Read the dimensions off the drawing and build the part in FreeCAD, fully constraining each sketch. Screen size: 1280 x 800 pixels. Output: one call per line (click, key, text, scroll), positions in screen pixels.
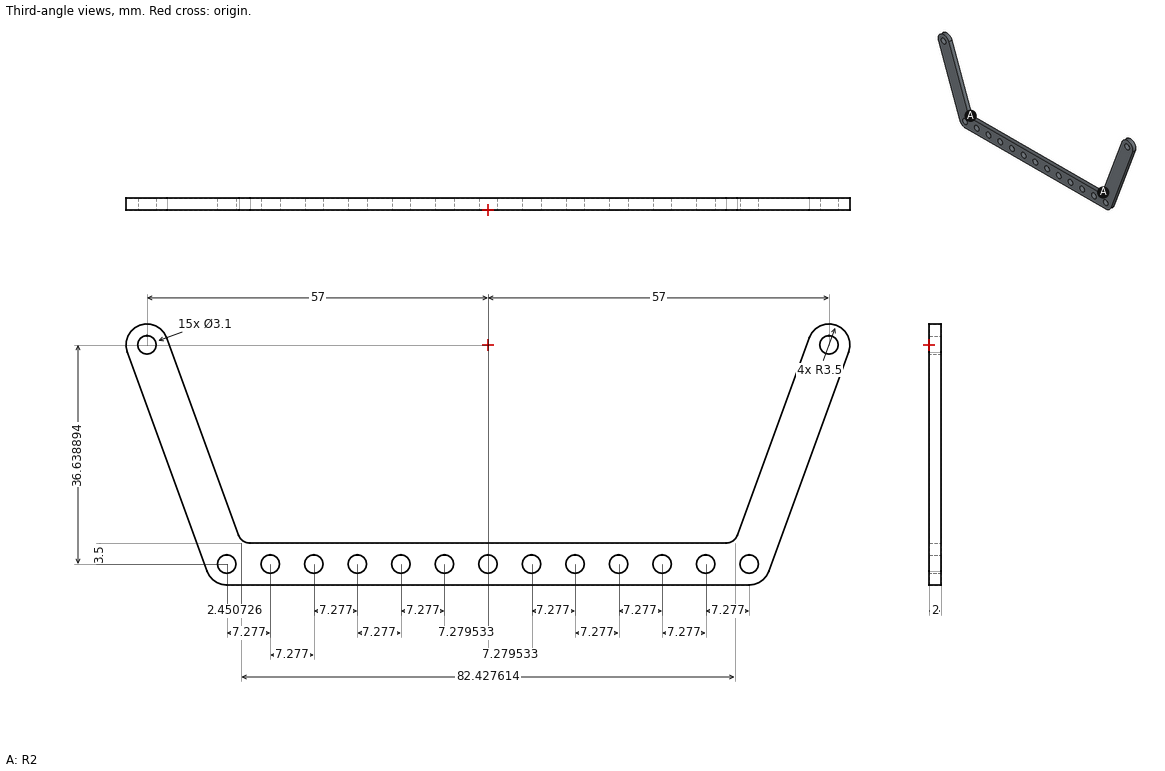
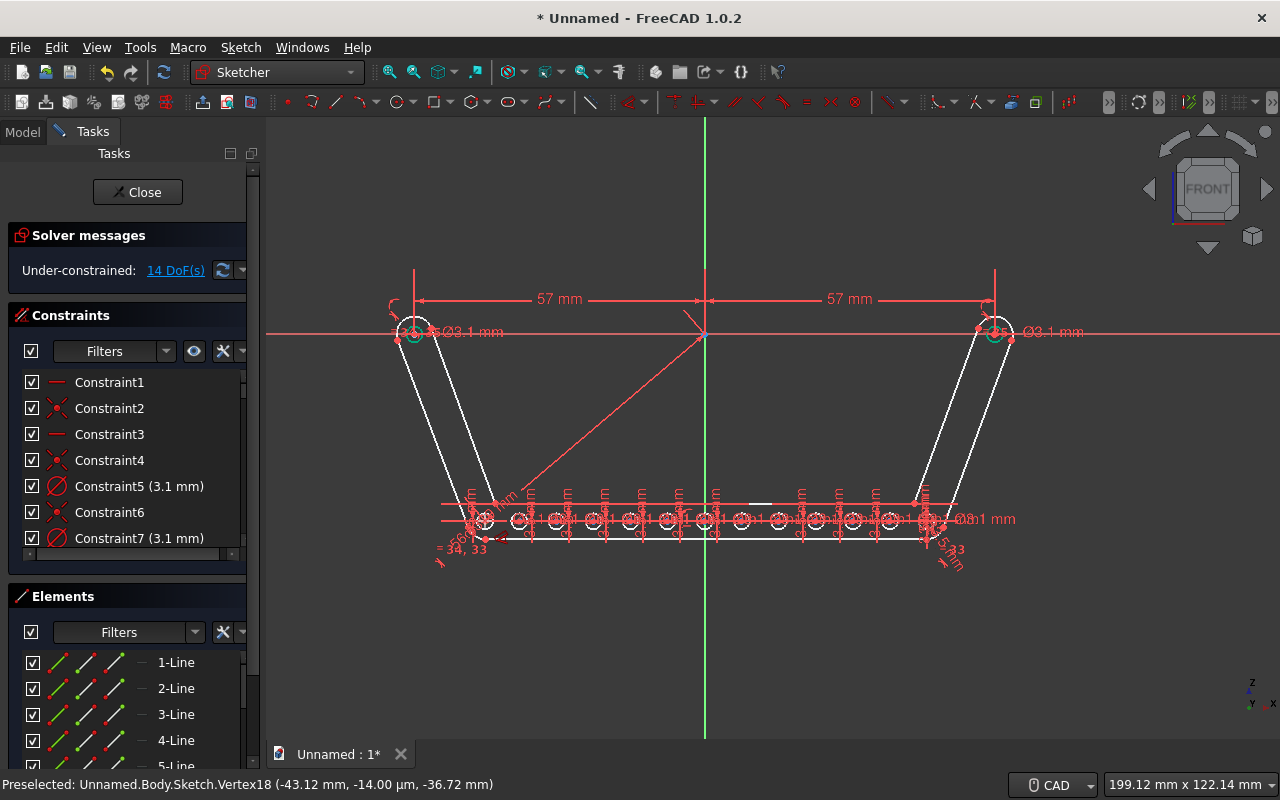
click(519, 521)
click(502, 555)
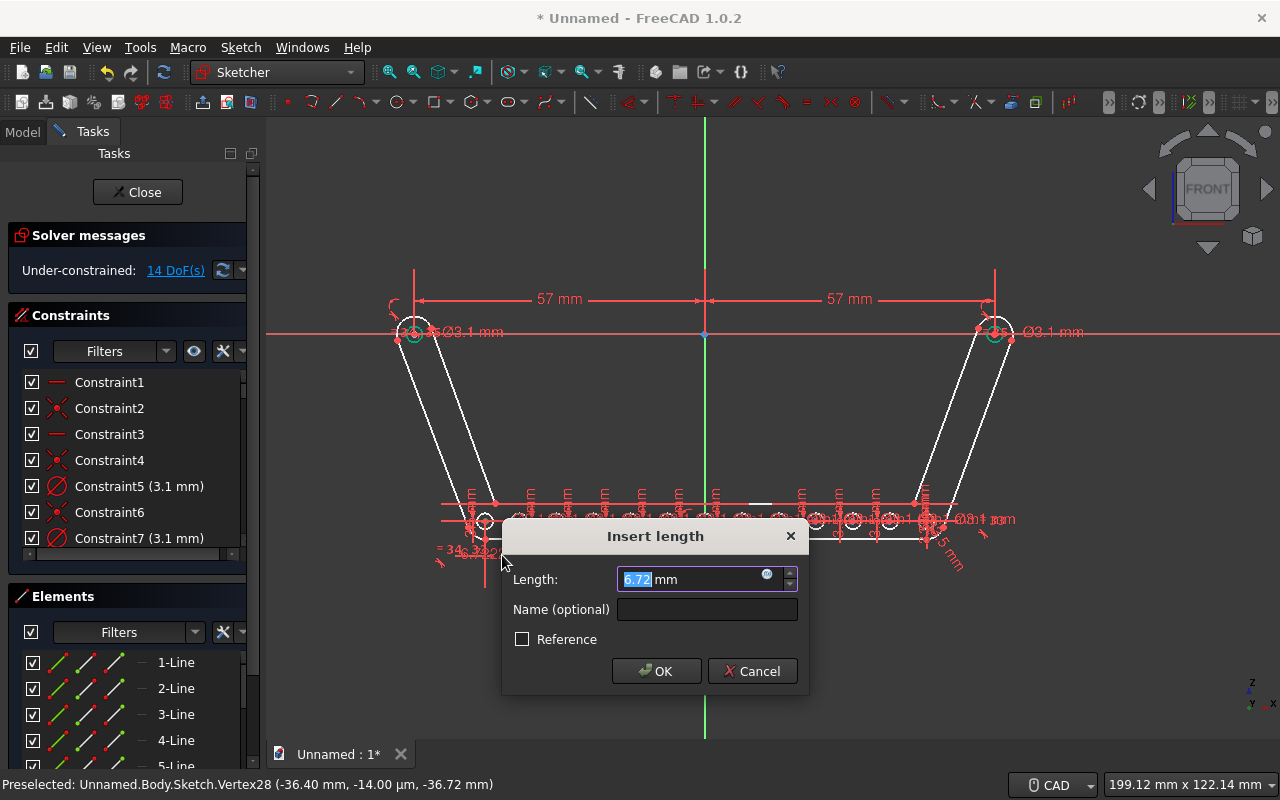
text(7.277)
key(Return)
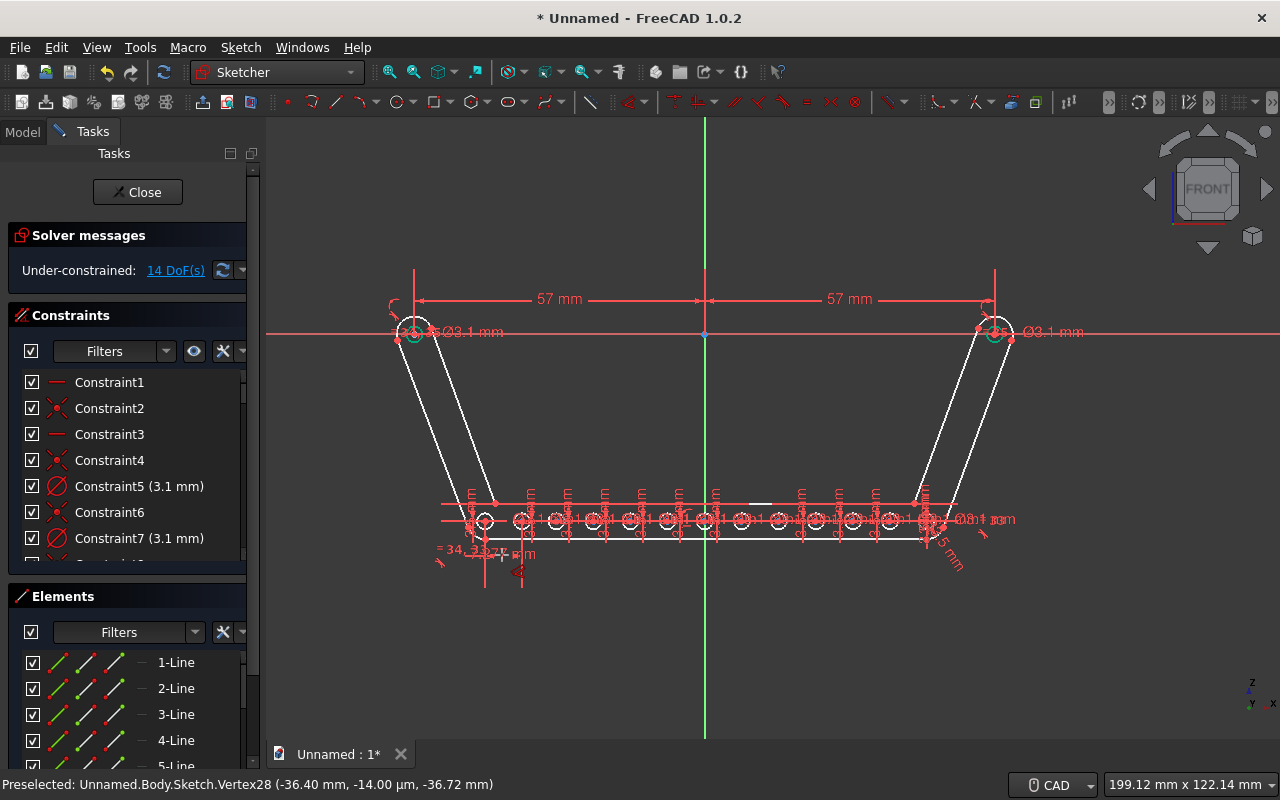
click(522, 521)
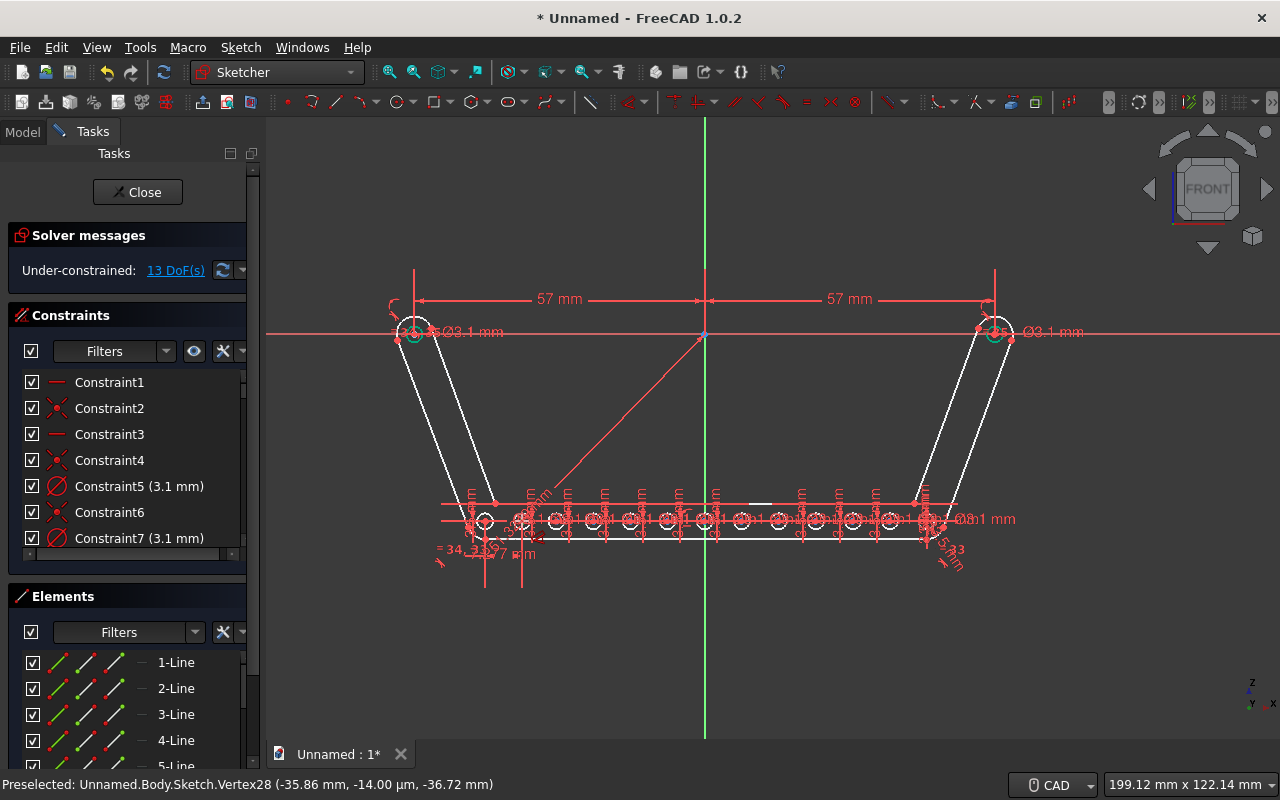
click(556, 521)
click(539, 487)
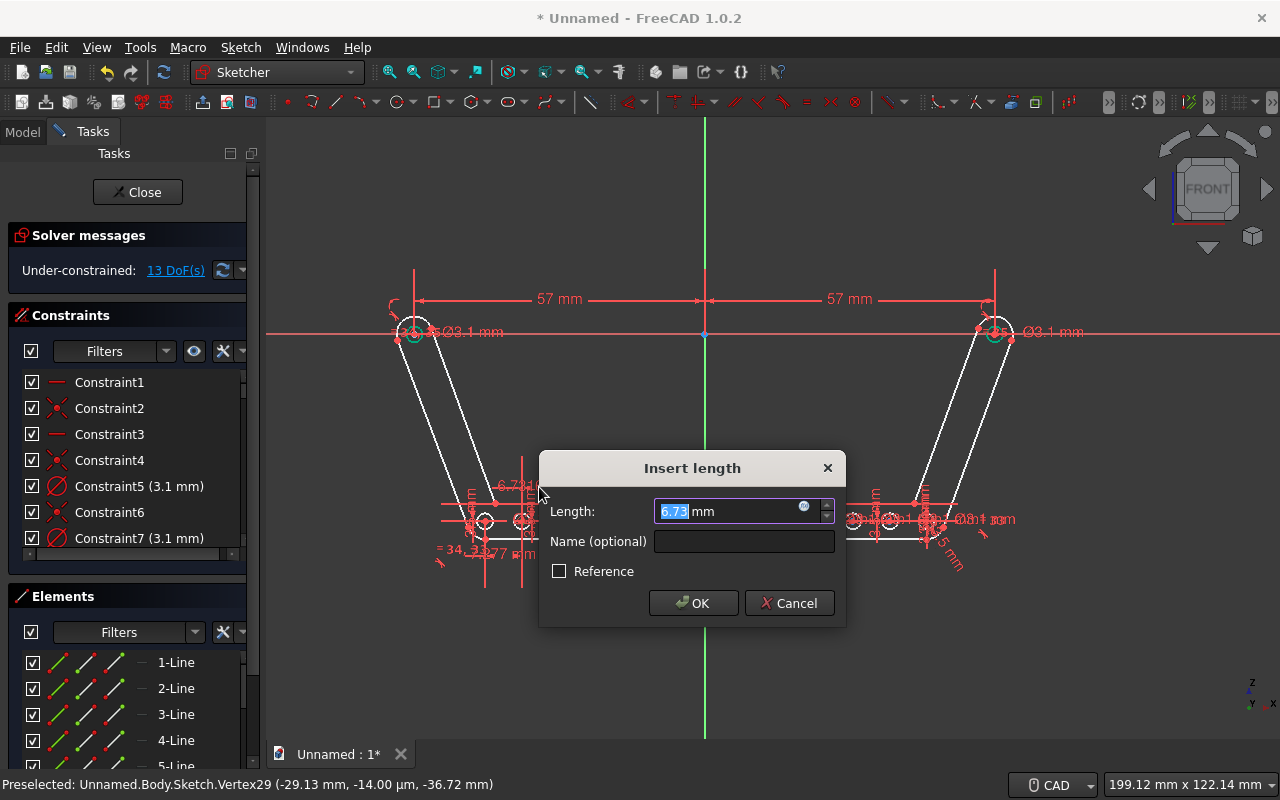
text(7.277)
key(Return)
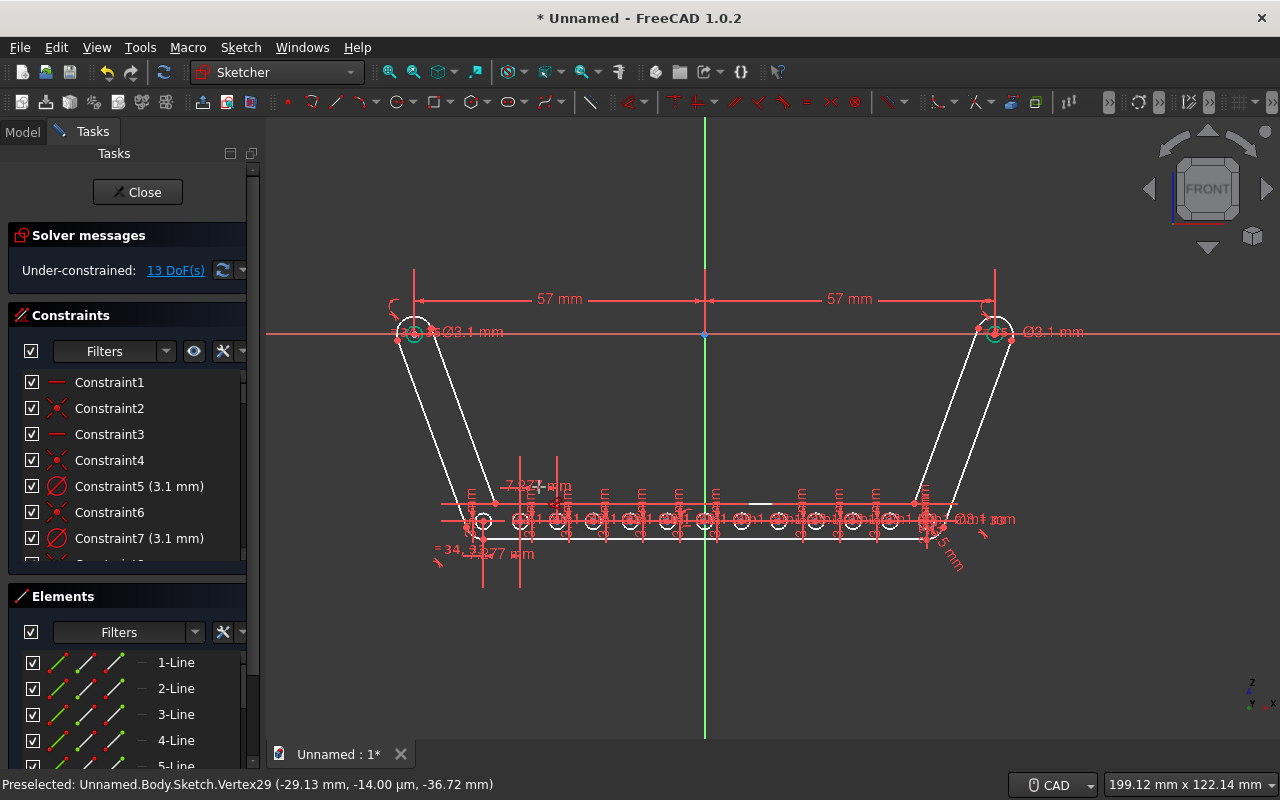
click(557, 521)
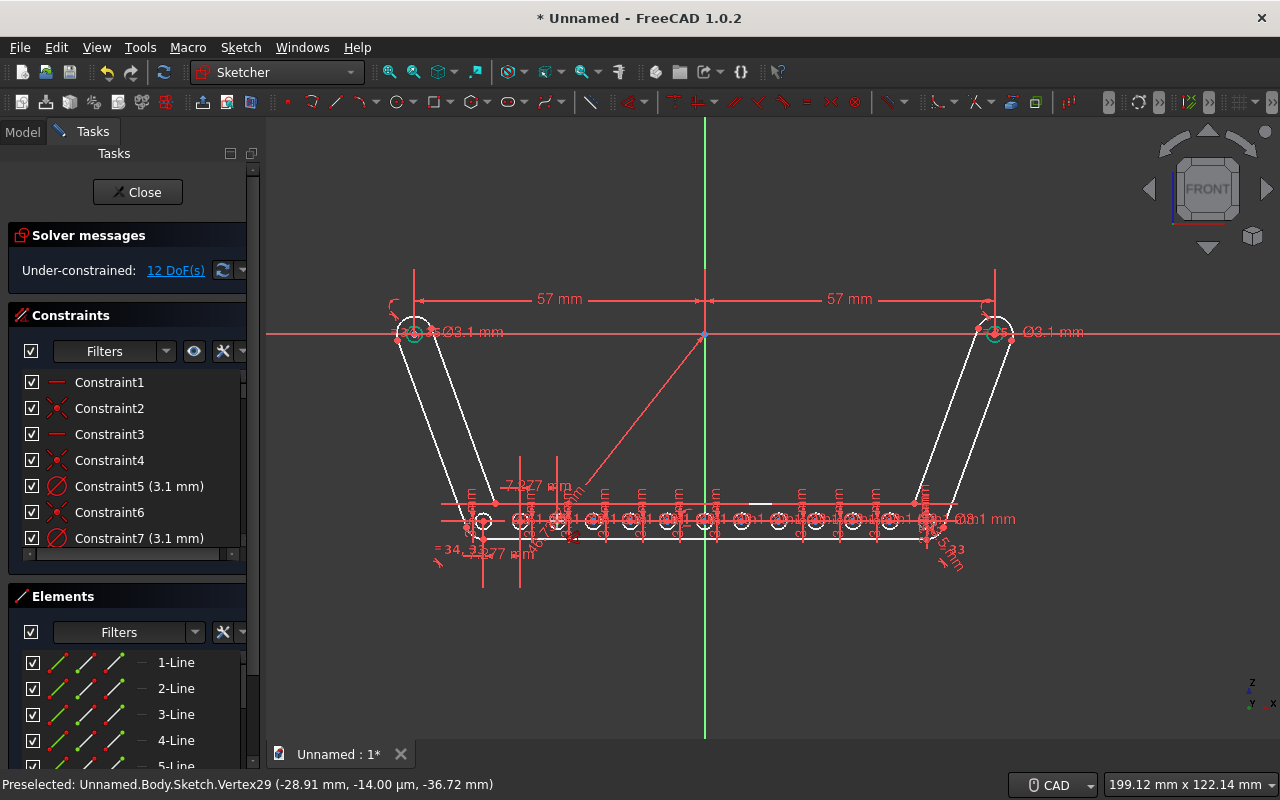
click(593, 521)
click(575, 555)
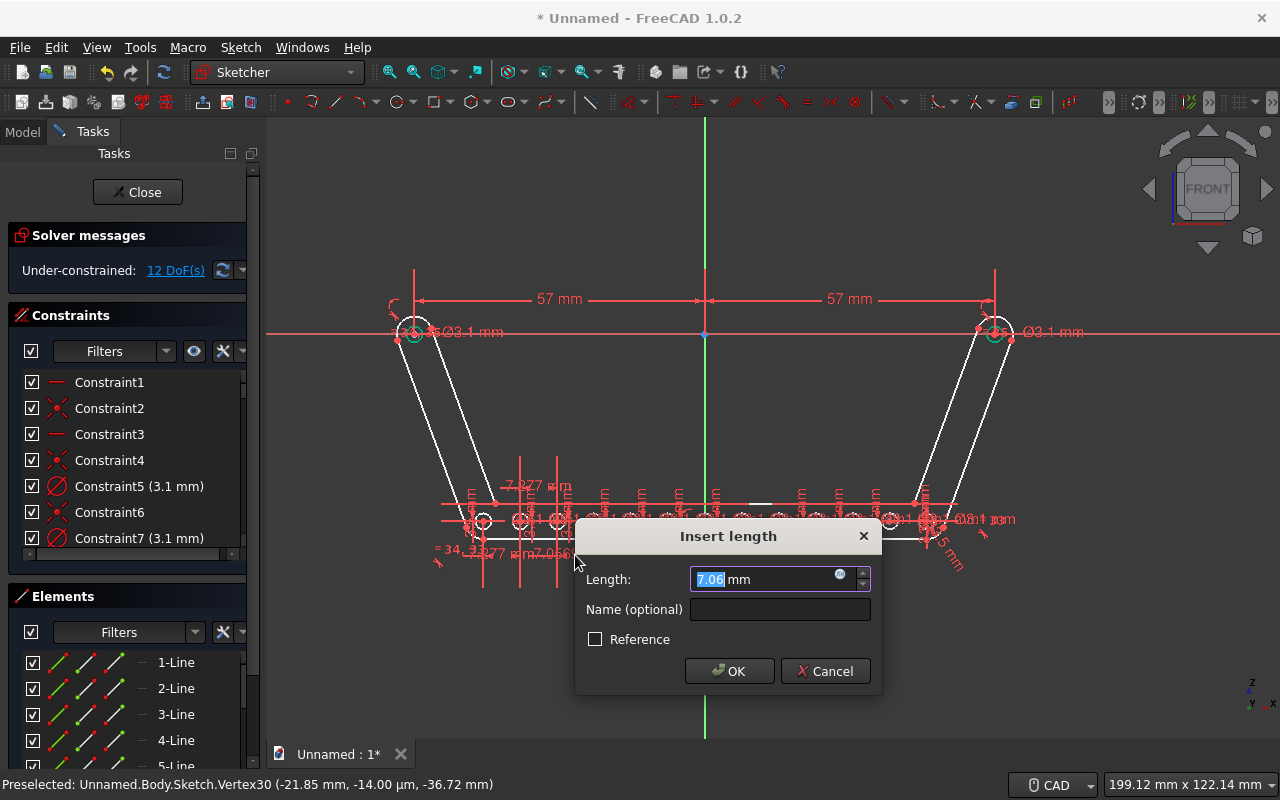
text(7.277)
key(Return)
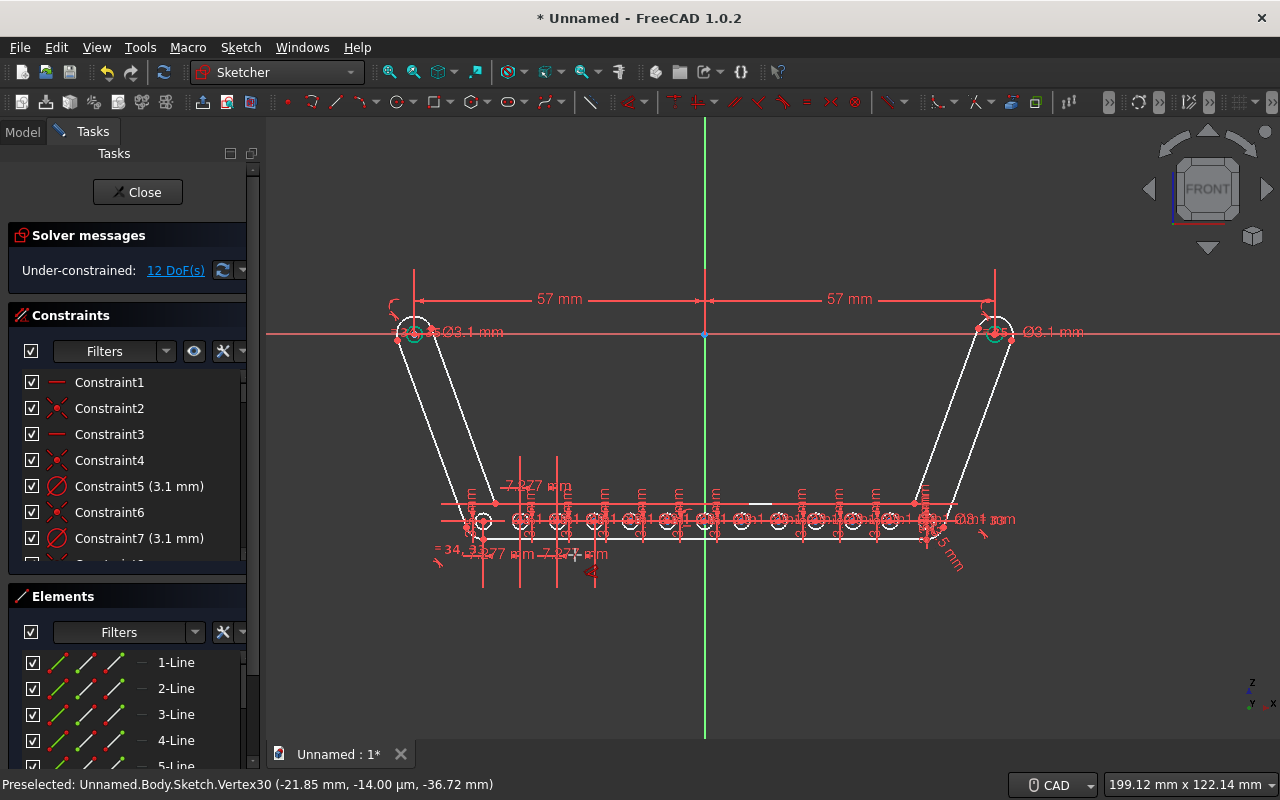
click(595, 521)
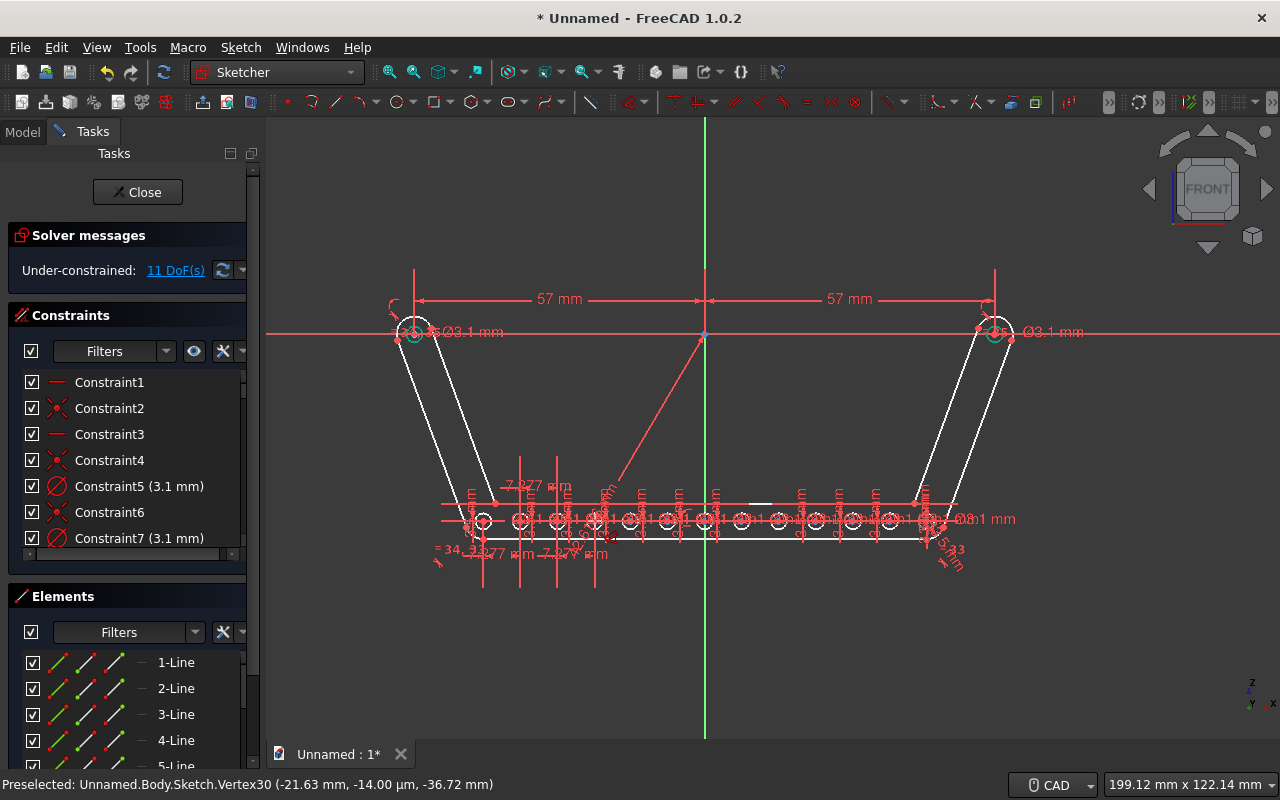
click(630, 521)
click(612, 487)